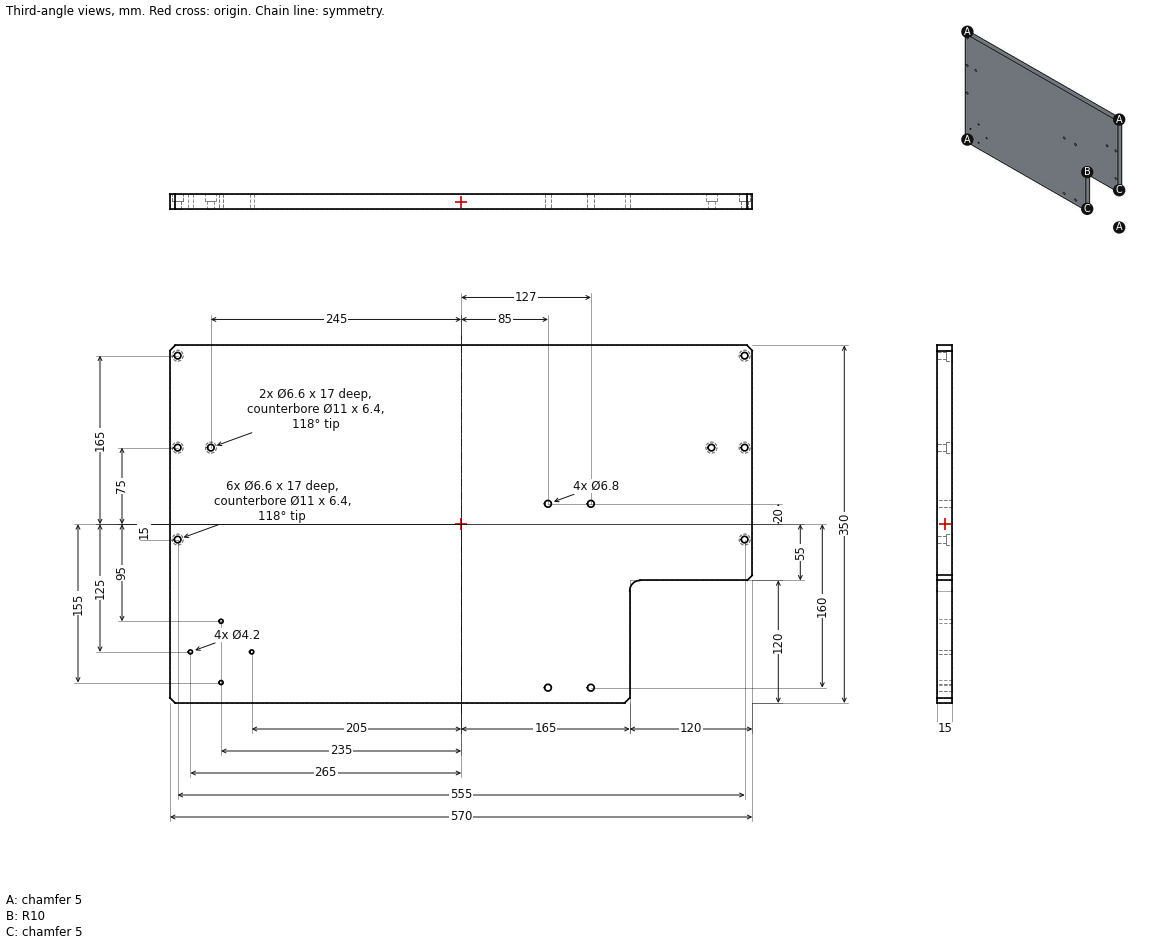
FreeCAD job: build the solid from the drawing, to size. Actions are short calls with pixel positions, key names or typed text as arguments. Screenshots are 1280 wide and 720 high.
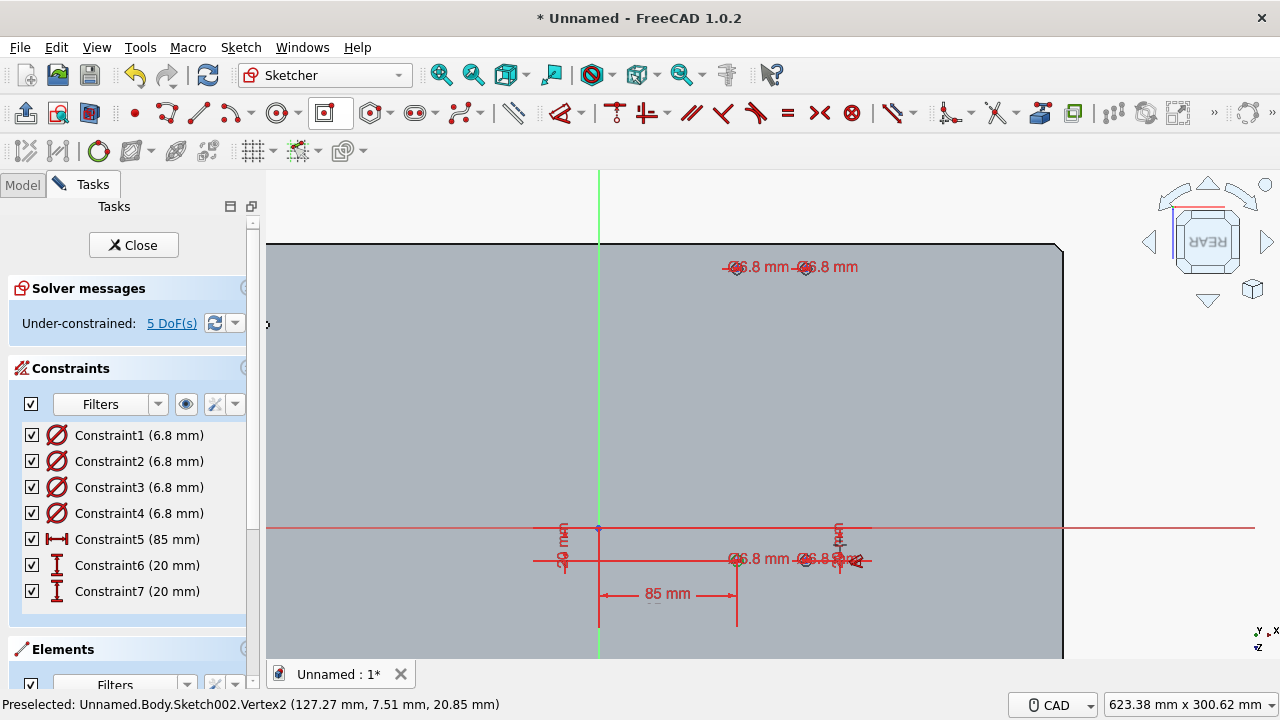
click(737, 269)
click(668, 235)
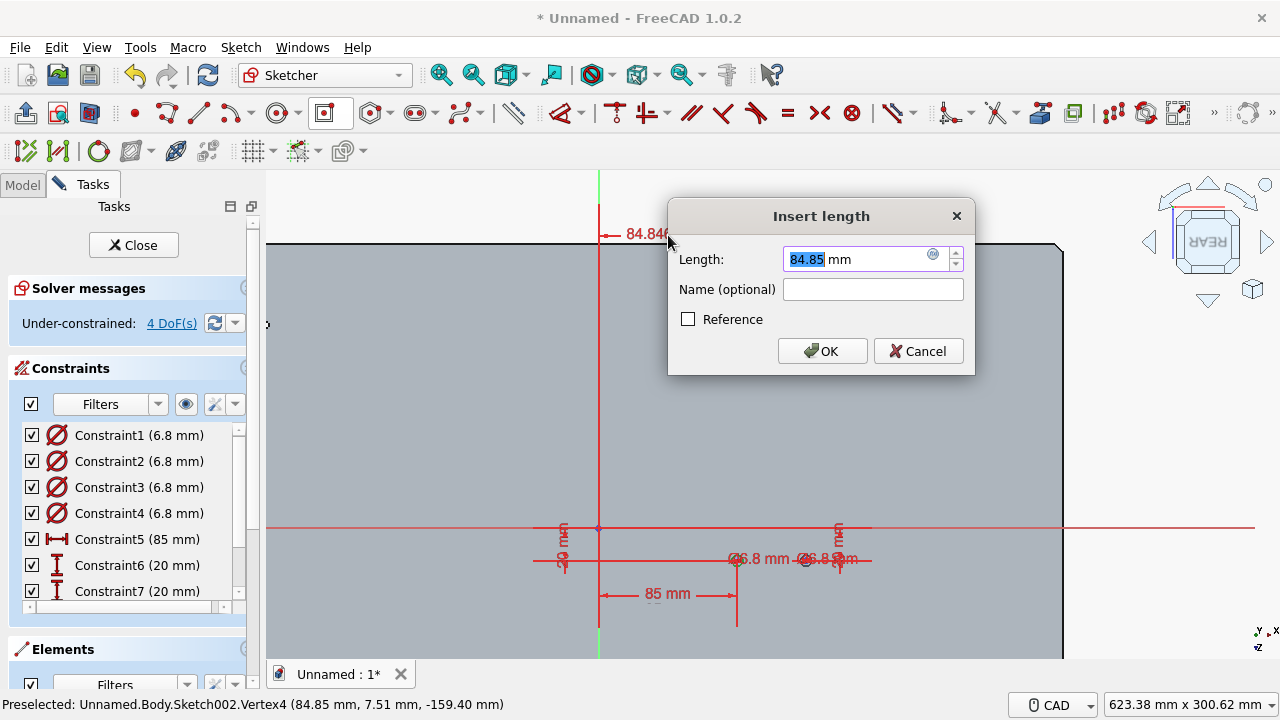
text(85)
key(Return)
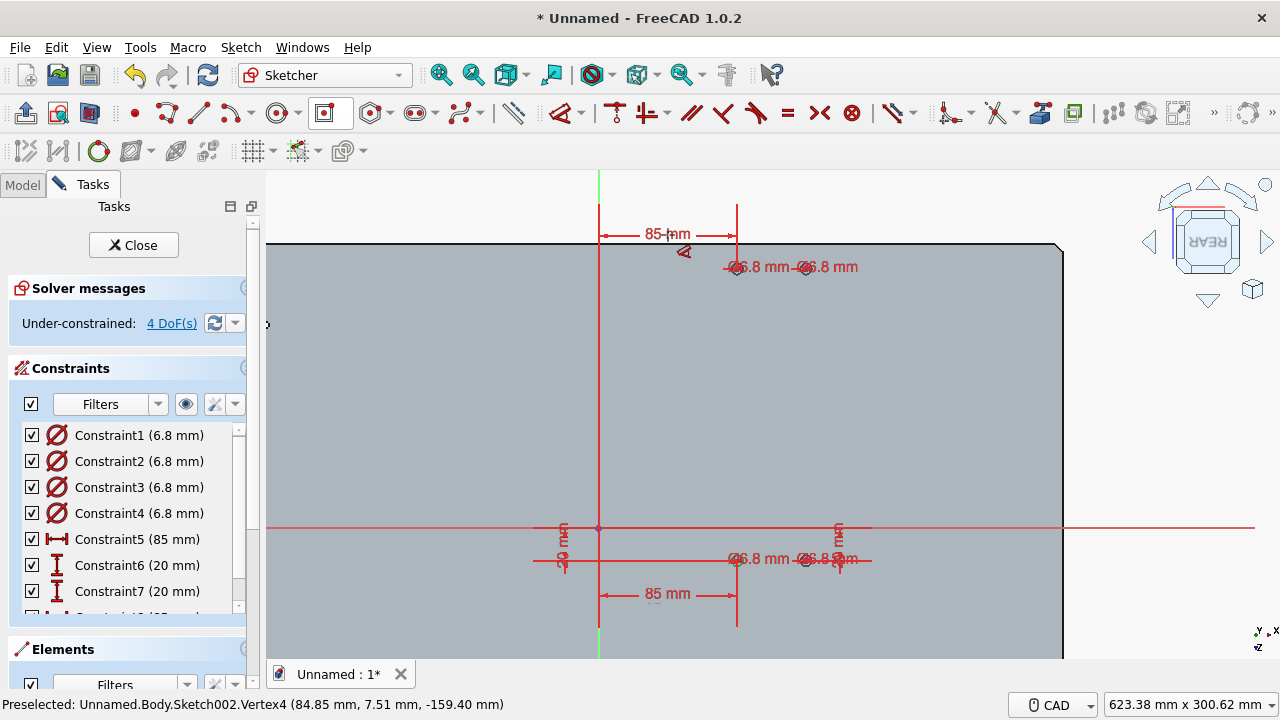
click(806, 561)
click(750, 595)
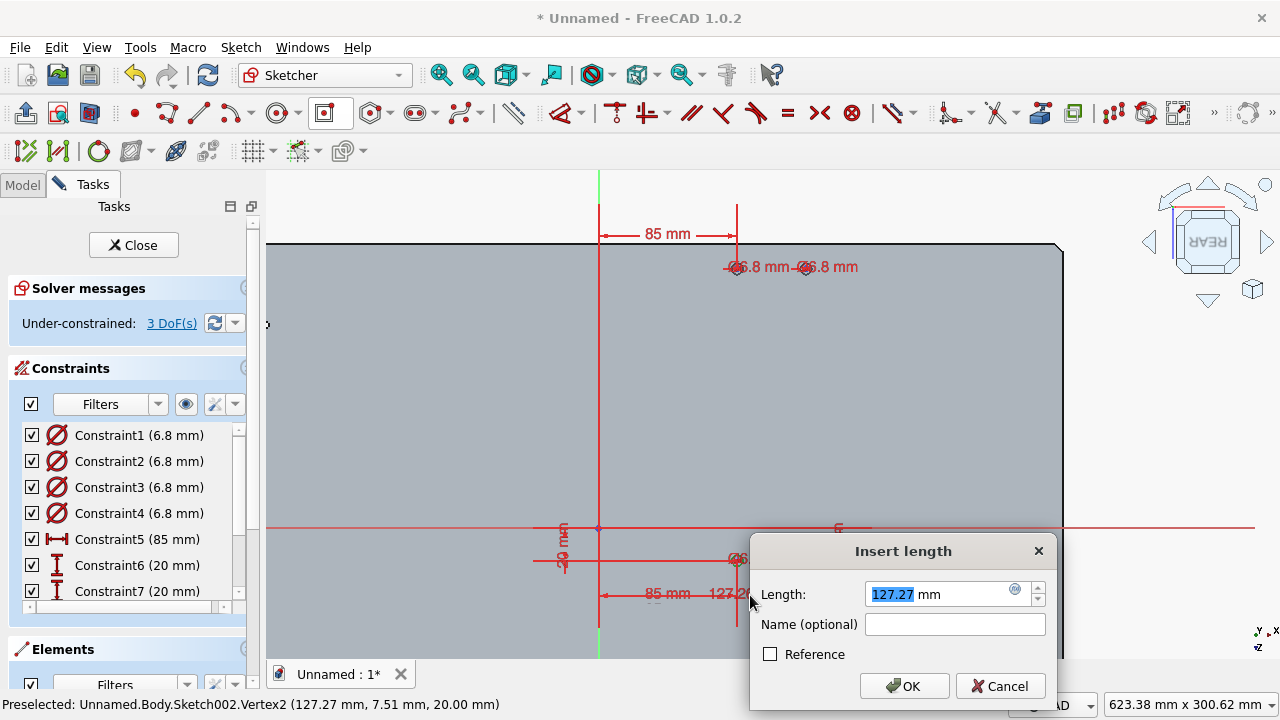
text(127)
key(Return)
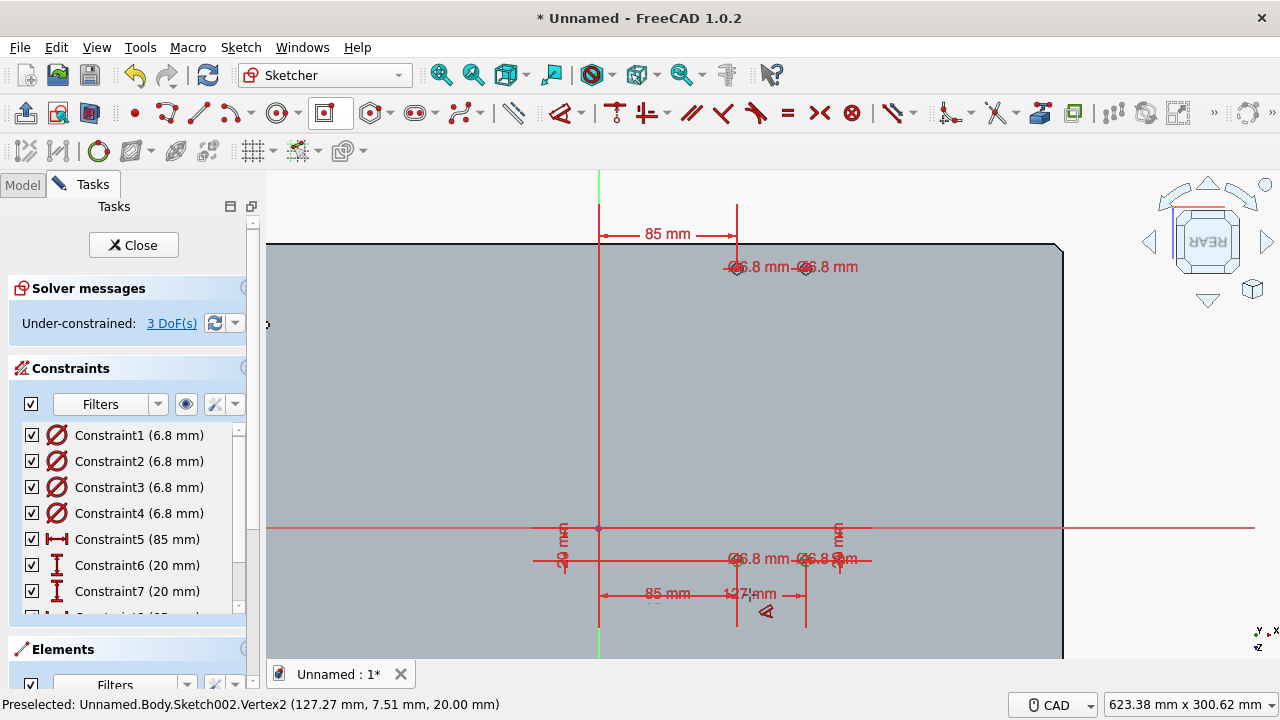
click(806, 269)
click(750, 235)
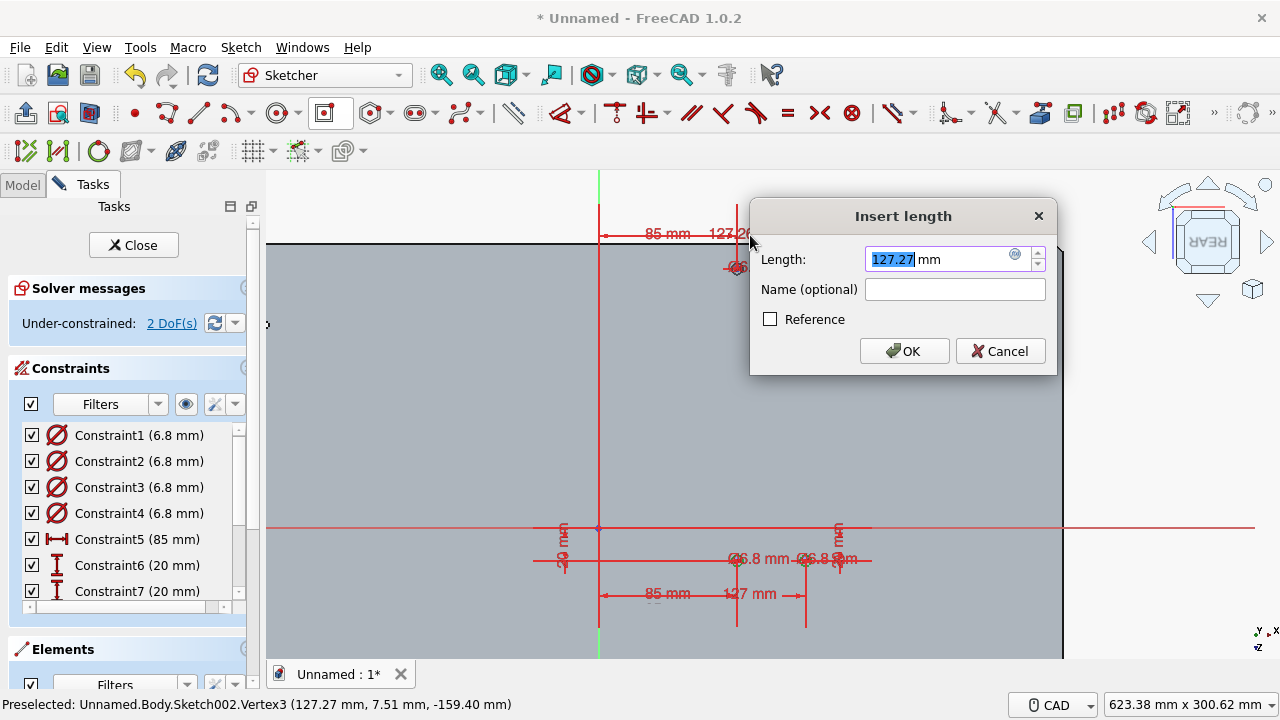
text(127)
key(Return)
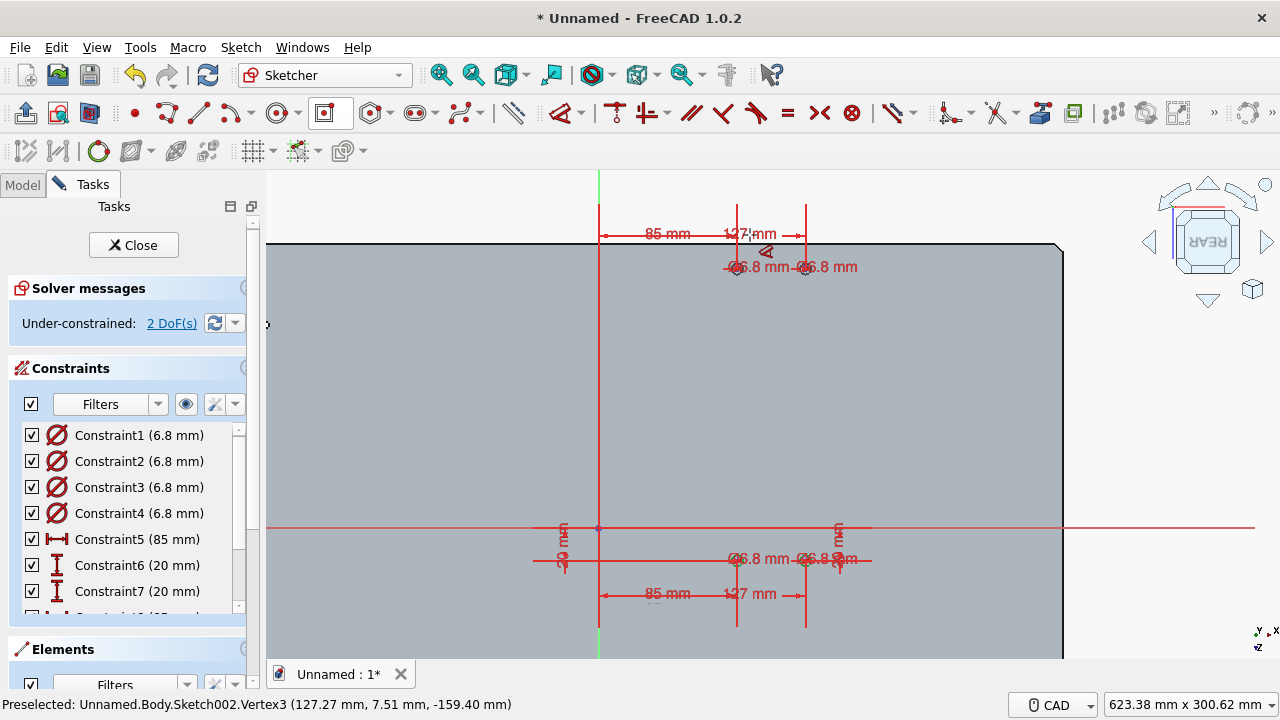
click(806, 269)
click(565, 399)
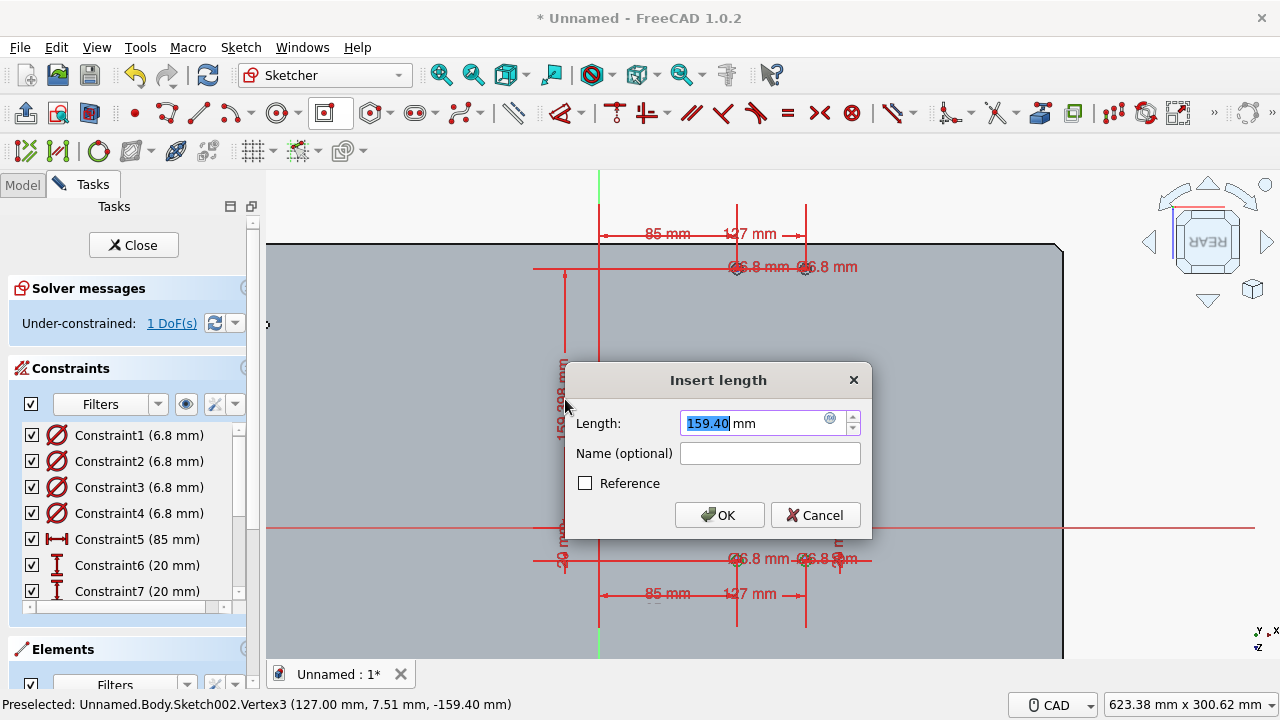
text(160)
key(Return)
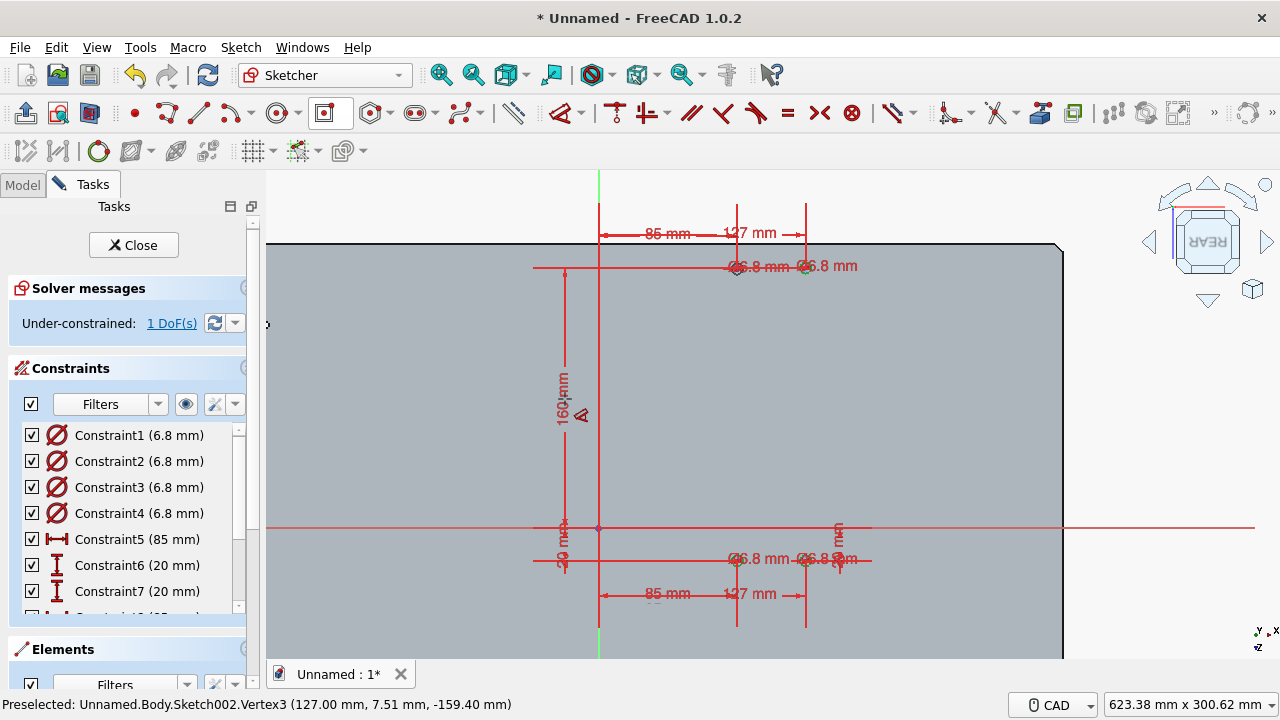
click(737, 269)
click(565, 339)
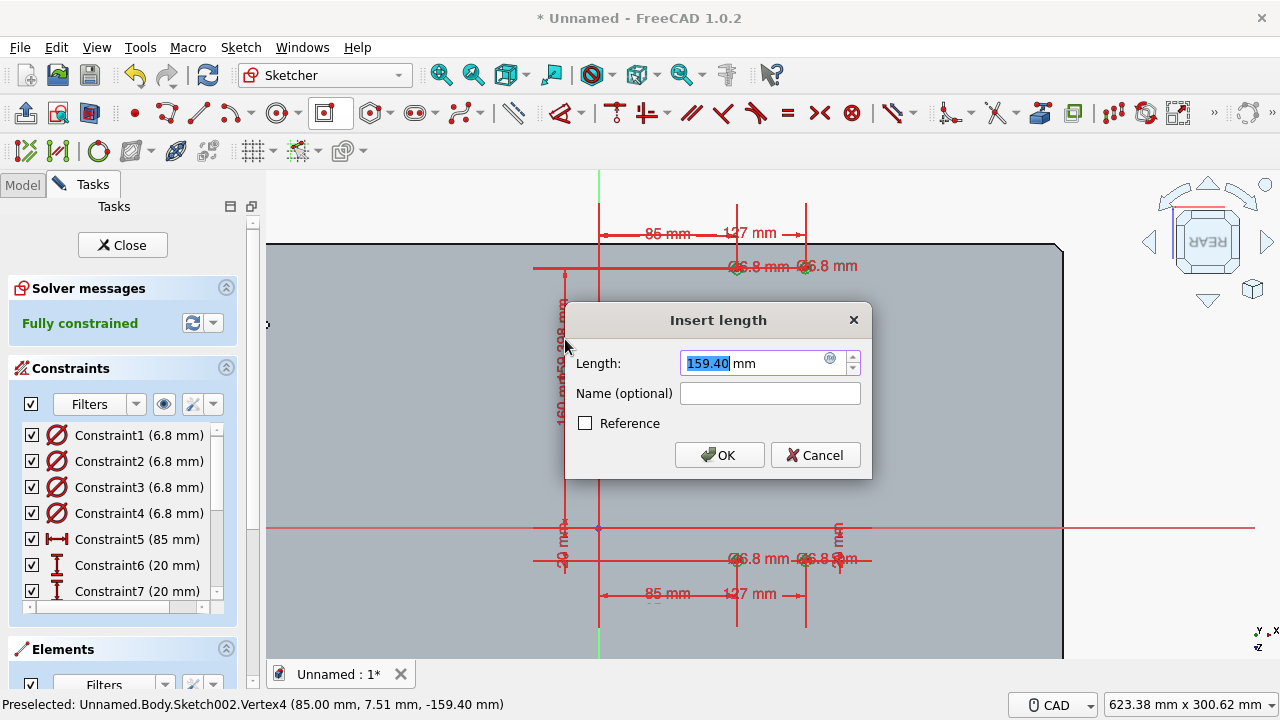
text(160)
key(Return)
key(Escape)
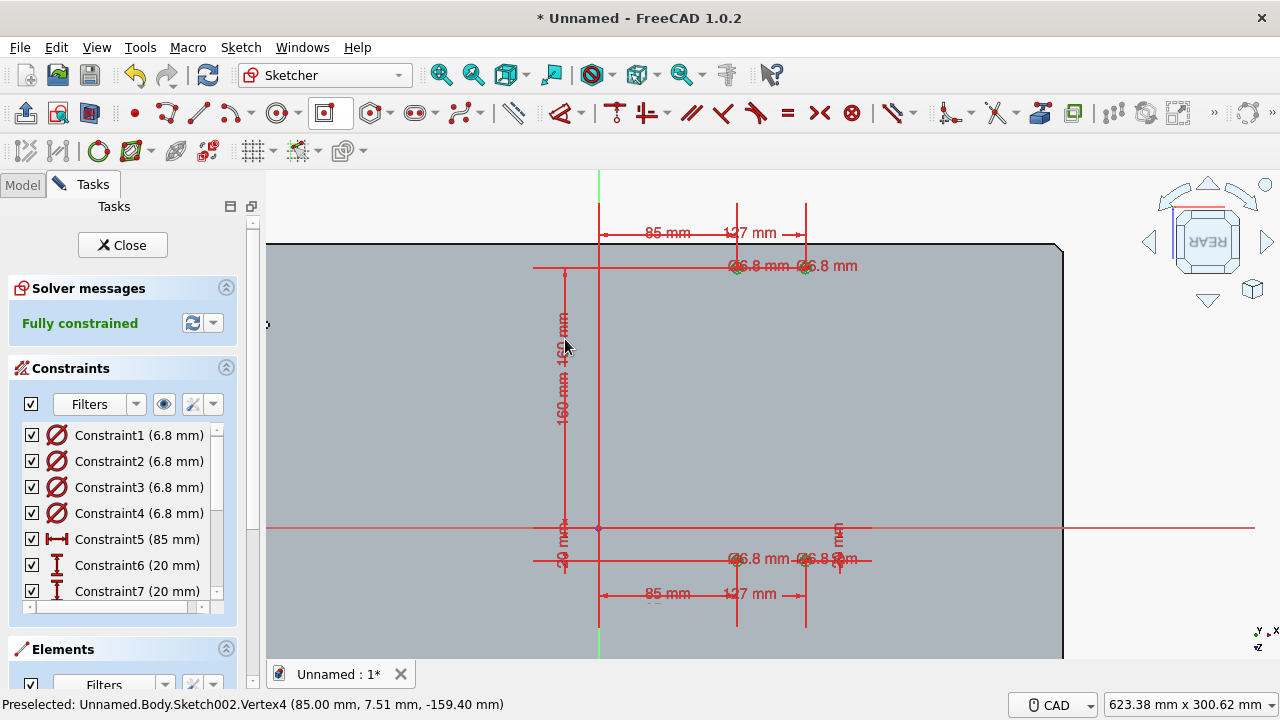
click(123, 245)